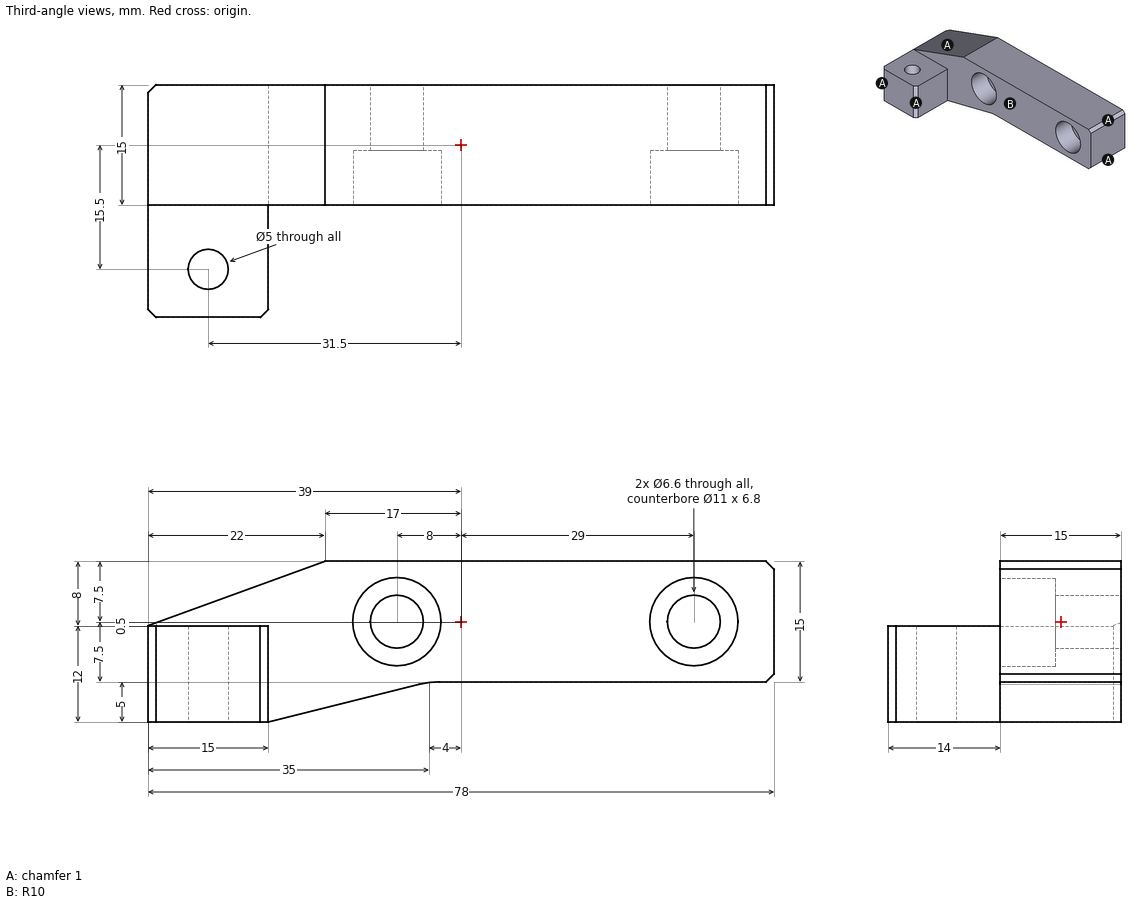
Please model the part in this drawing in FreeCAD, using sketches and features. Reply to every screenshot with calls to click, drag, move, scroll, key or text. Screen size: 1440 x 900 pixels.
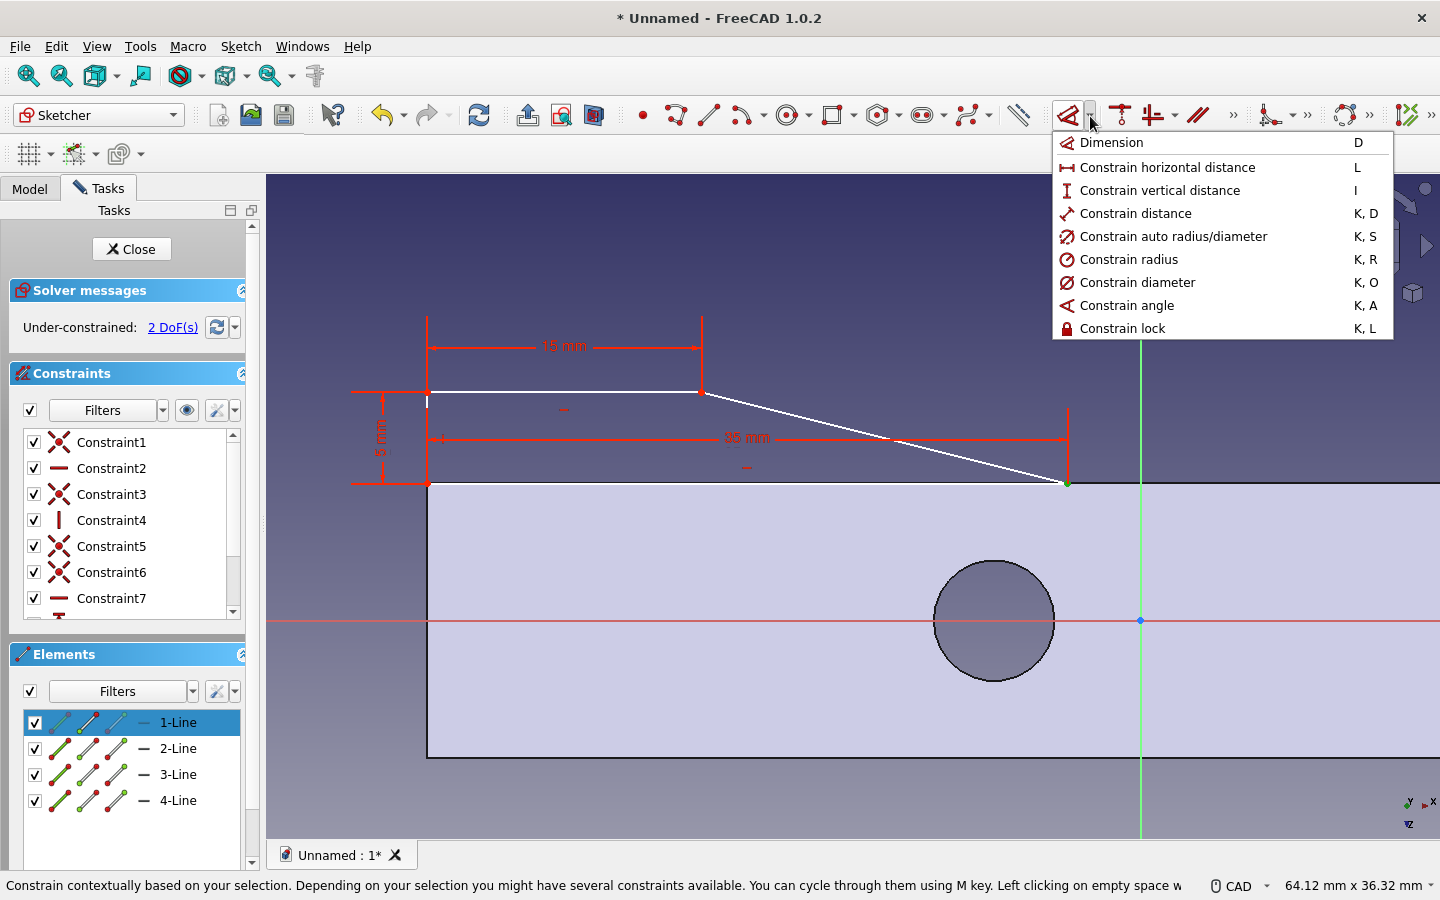
click(1223, 168)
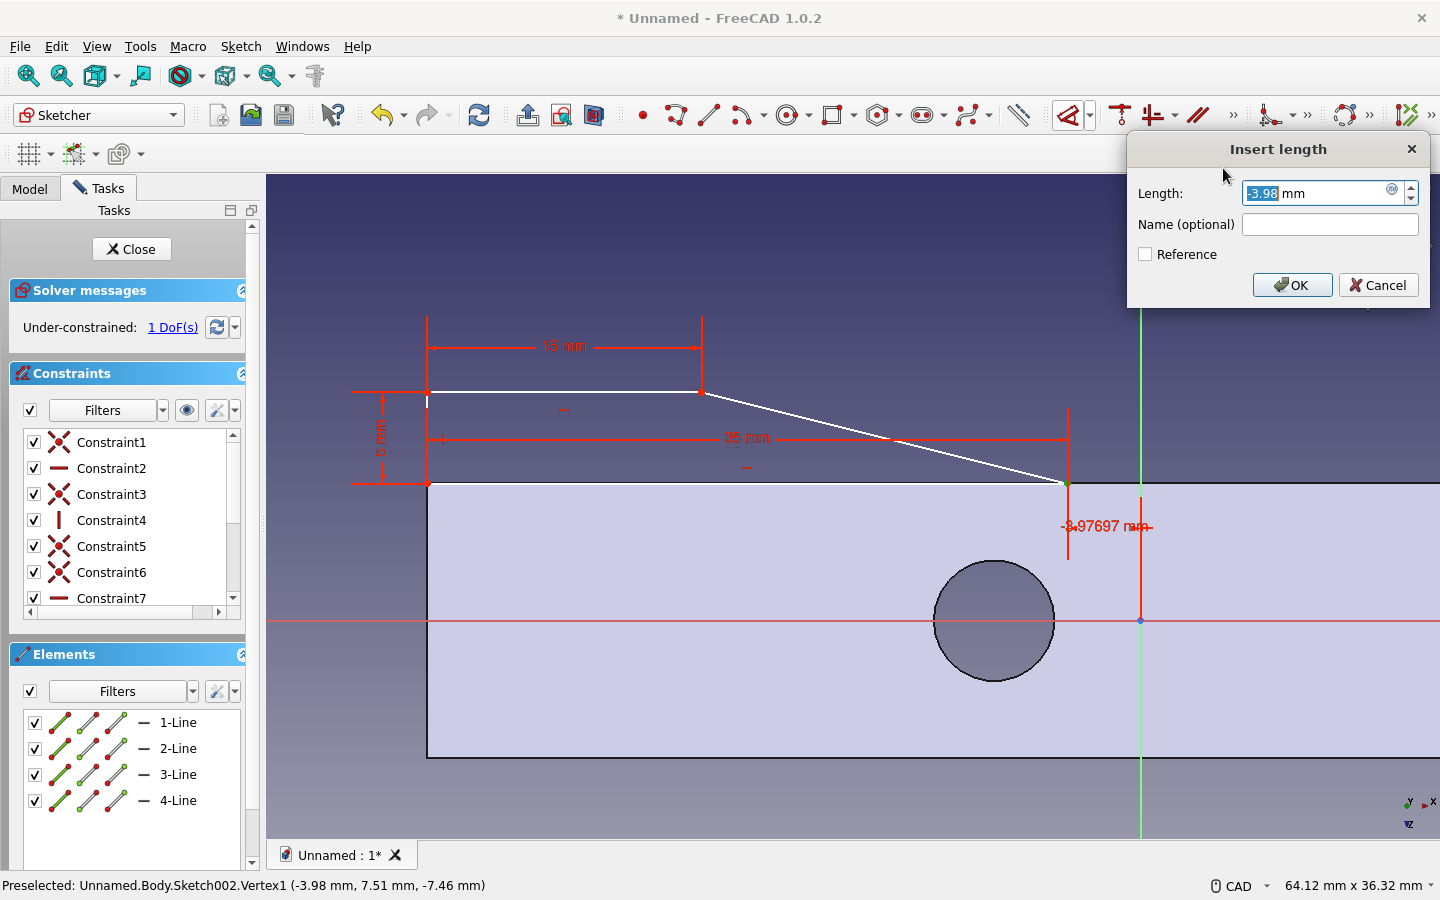
text(-4)
key(Return)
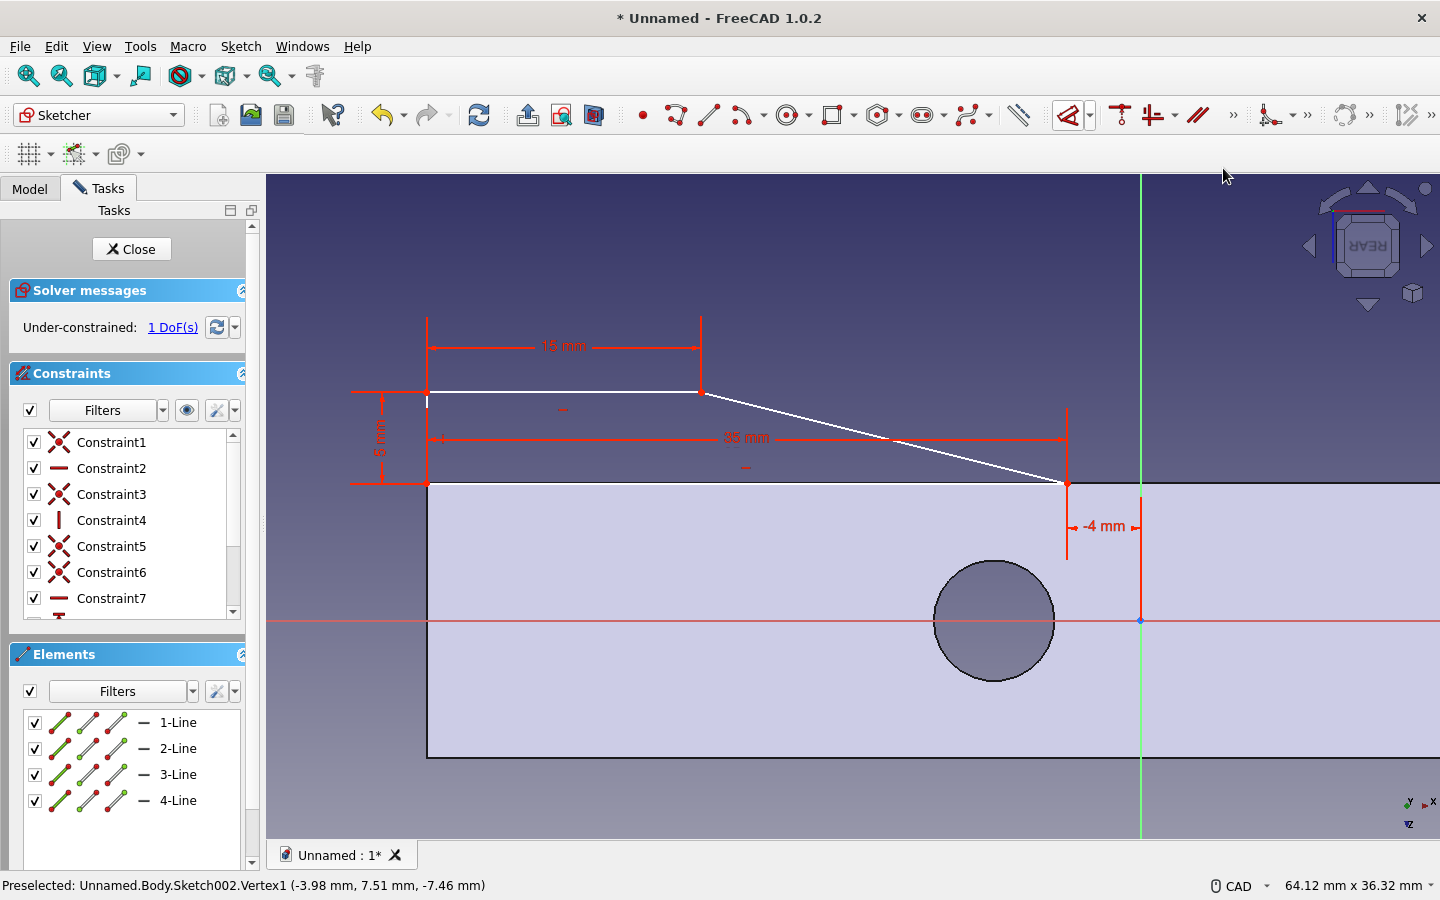
click(1067, 484)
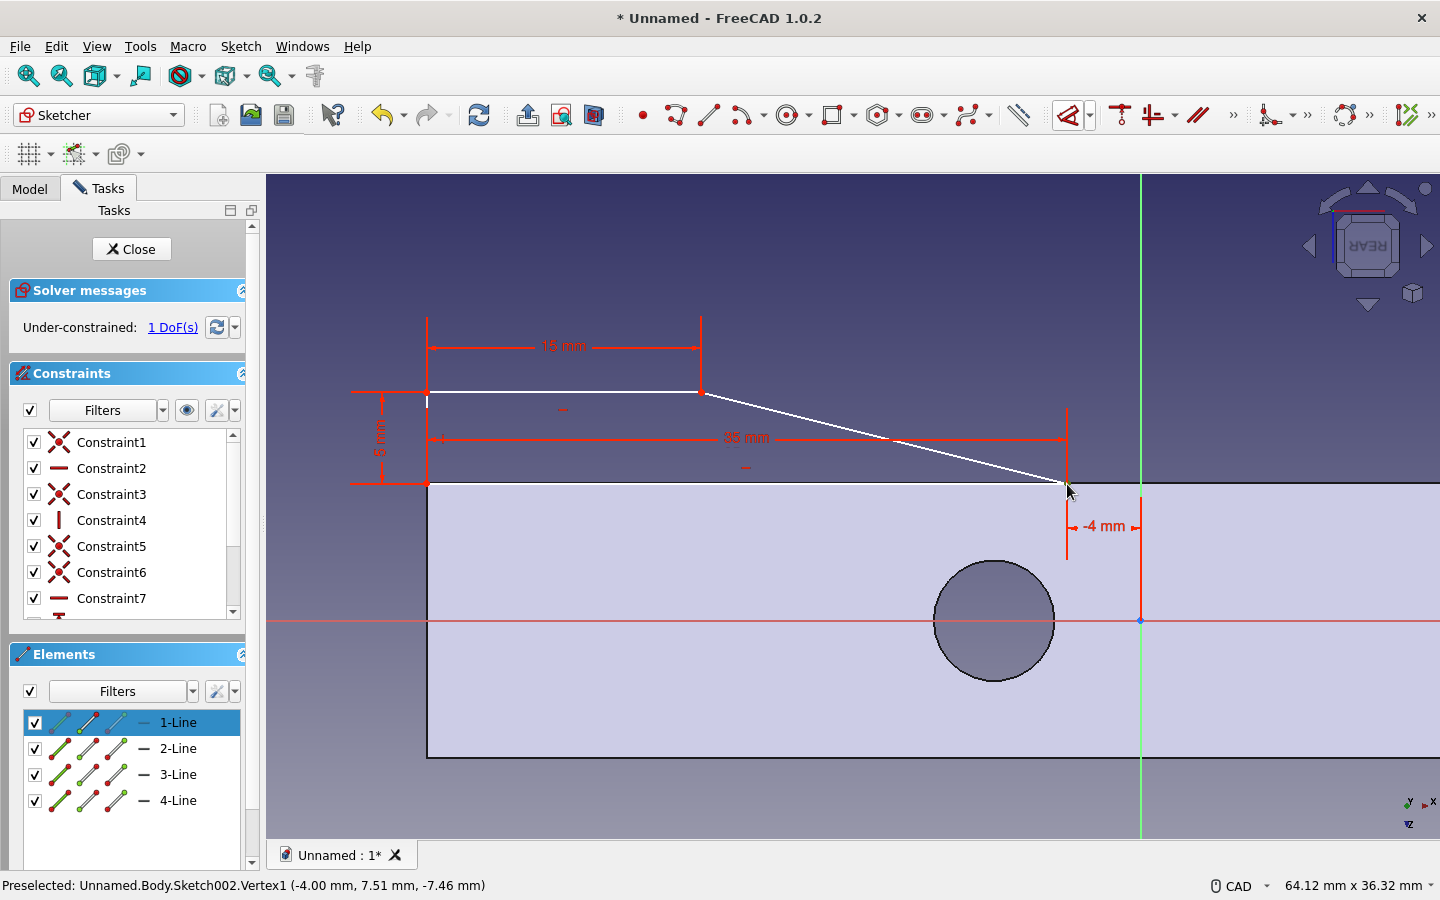
click(1090, 116)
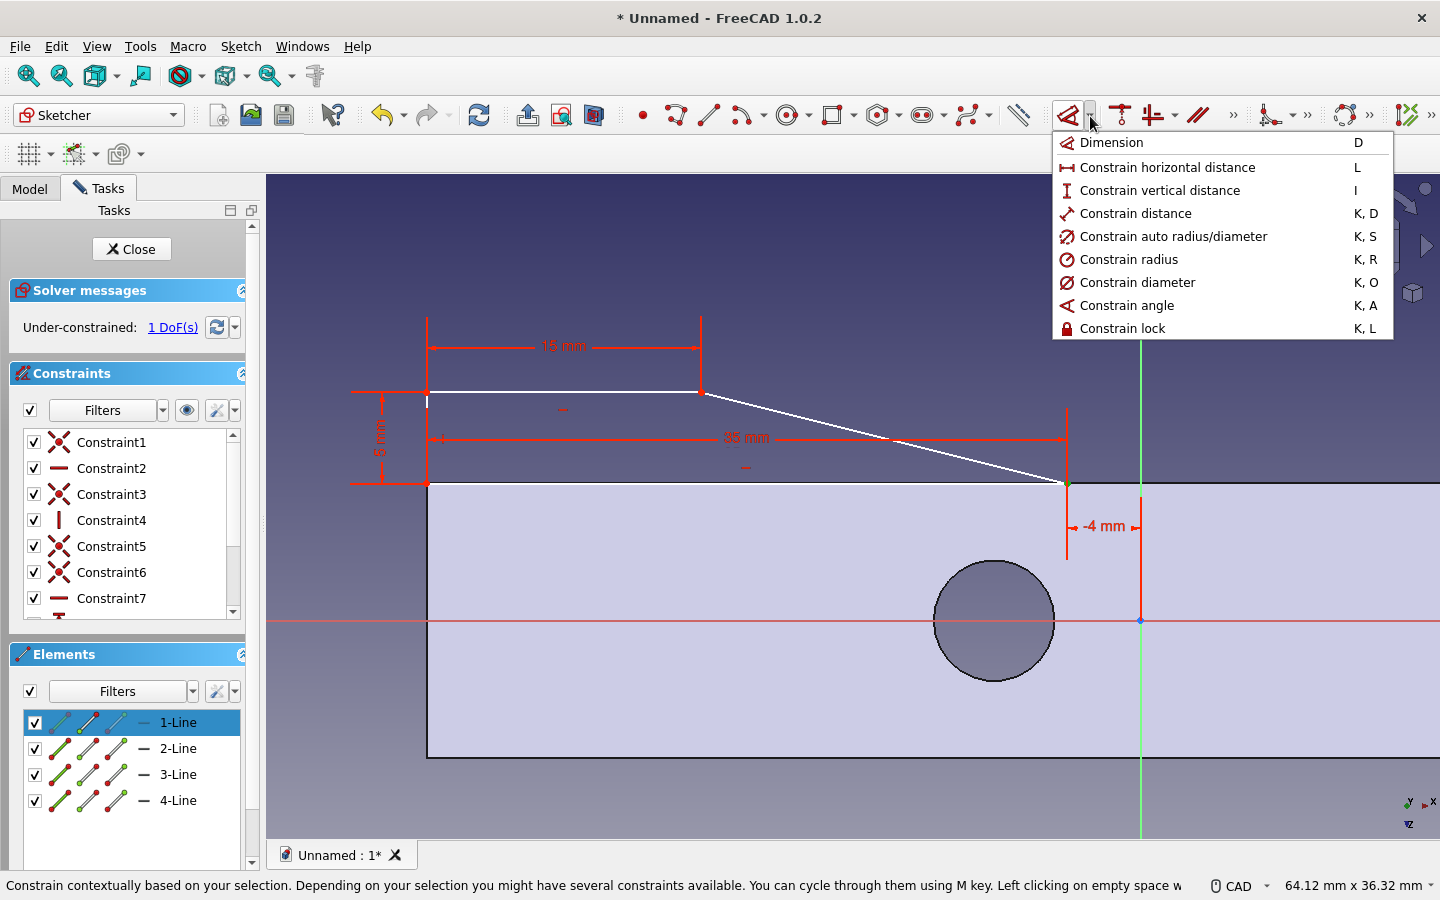
click(1223, 190)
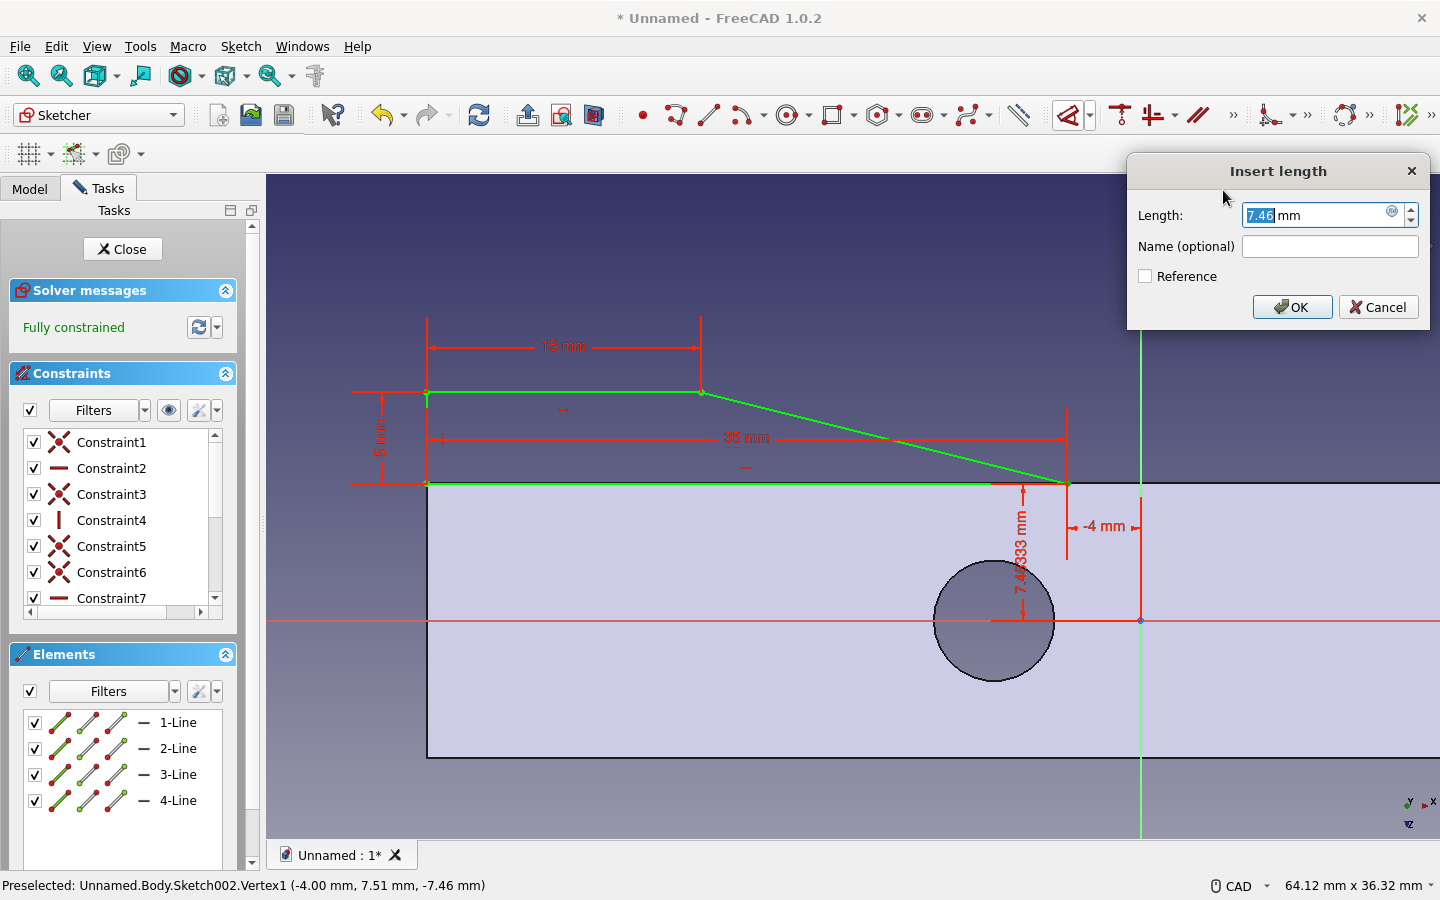
text(7.5)
key(Return)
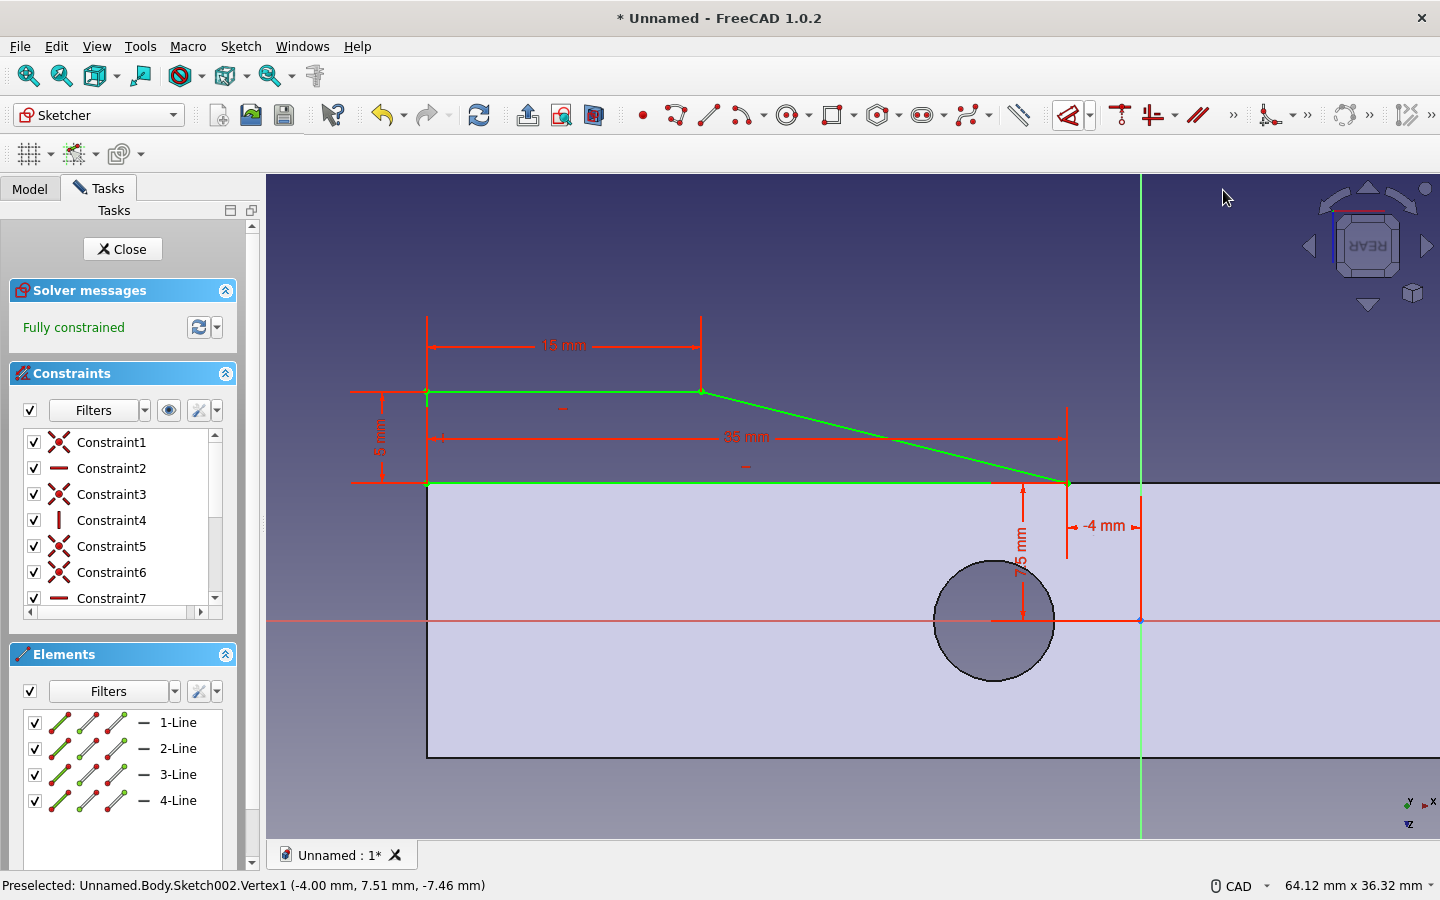
click(123, 249)